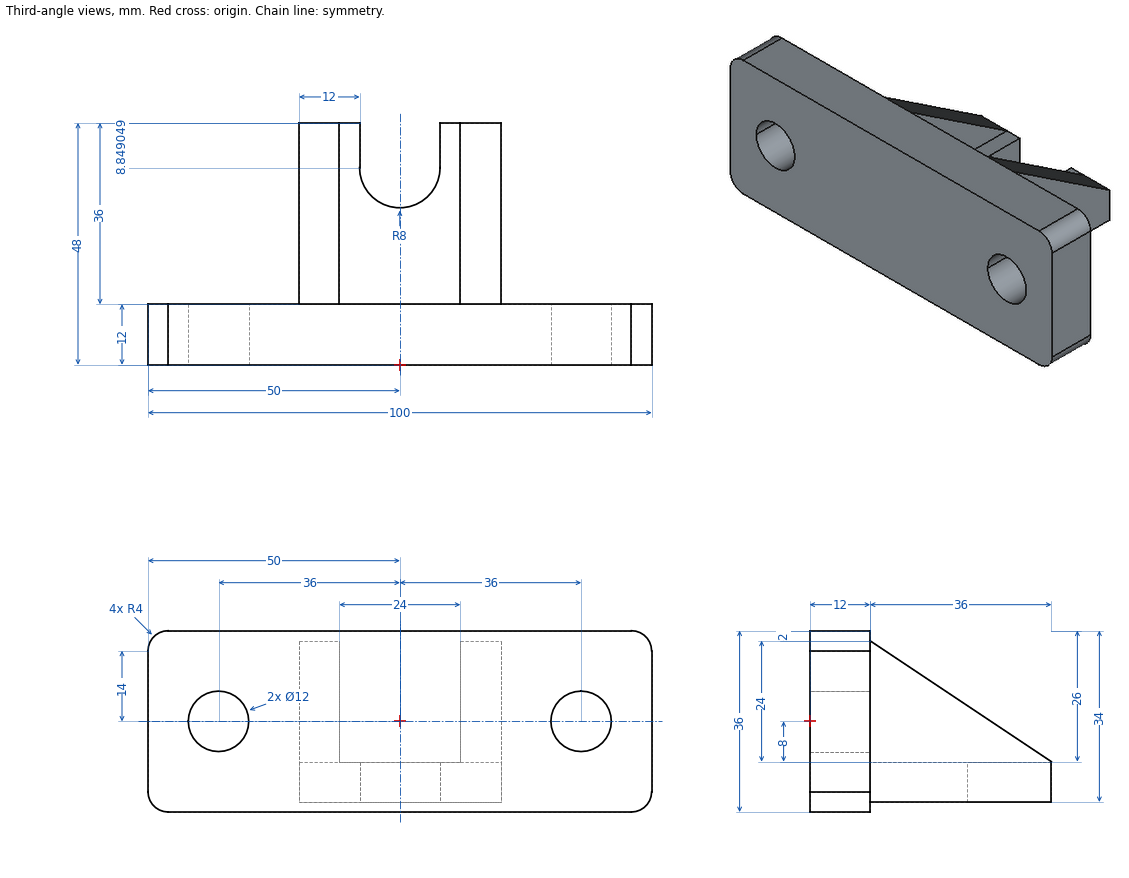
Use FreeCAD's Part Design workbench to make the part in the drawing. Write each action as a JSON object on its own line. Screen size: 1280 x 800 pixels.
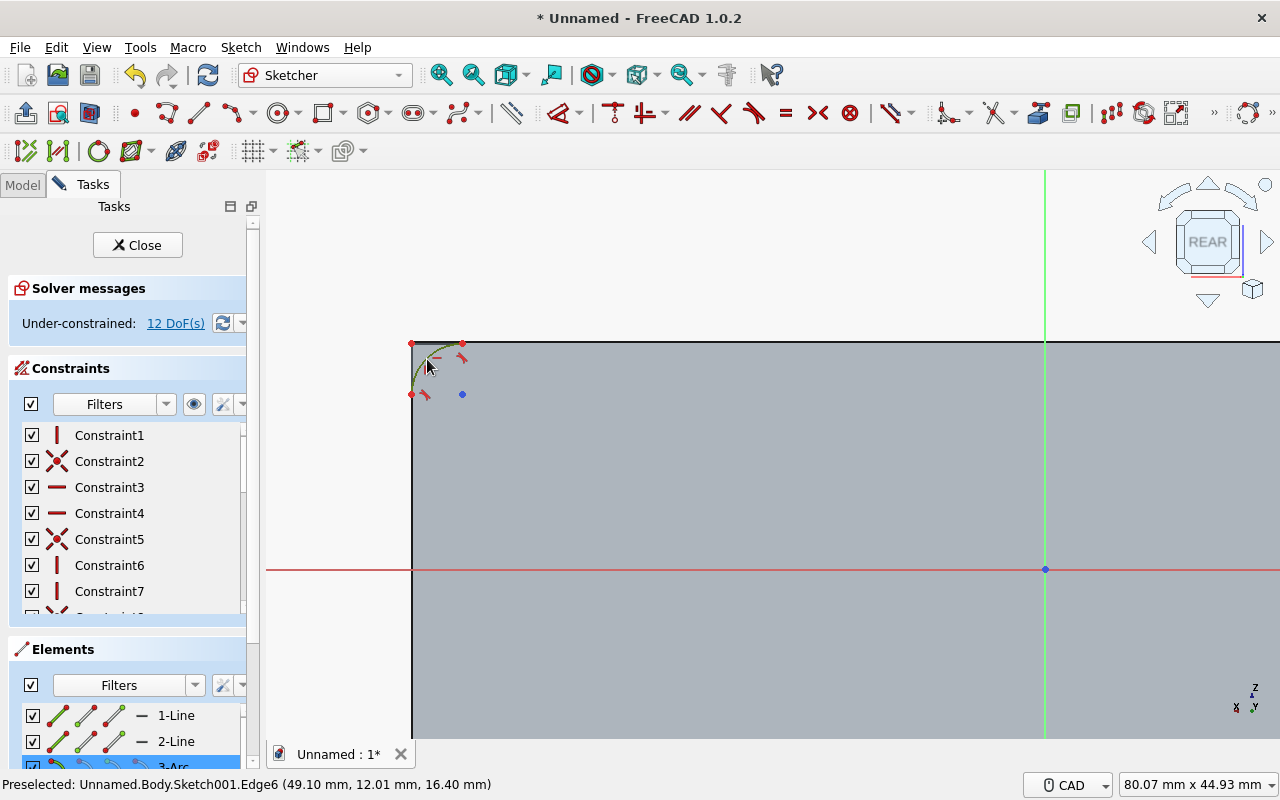
{"action": "scroll", "coordinate": [426, 360], "scroll_direction": "down", "scroll_amount": 4}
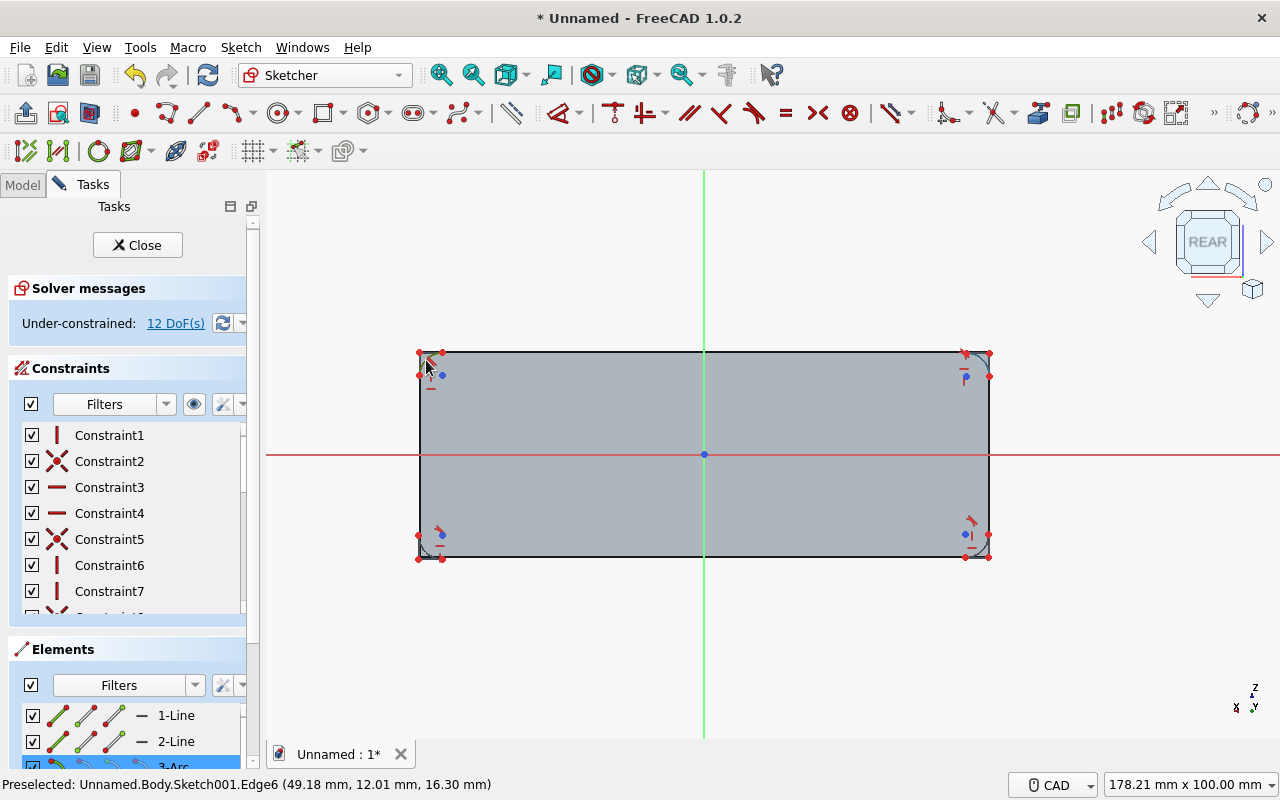
{"action": "scroll", "coordinate": [426, 552], "scroll_direction": "up", "scroll_amount": 4}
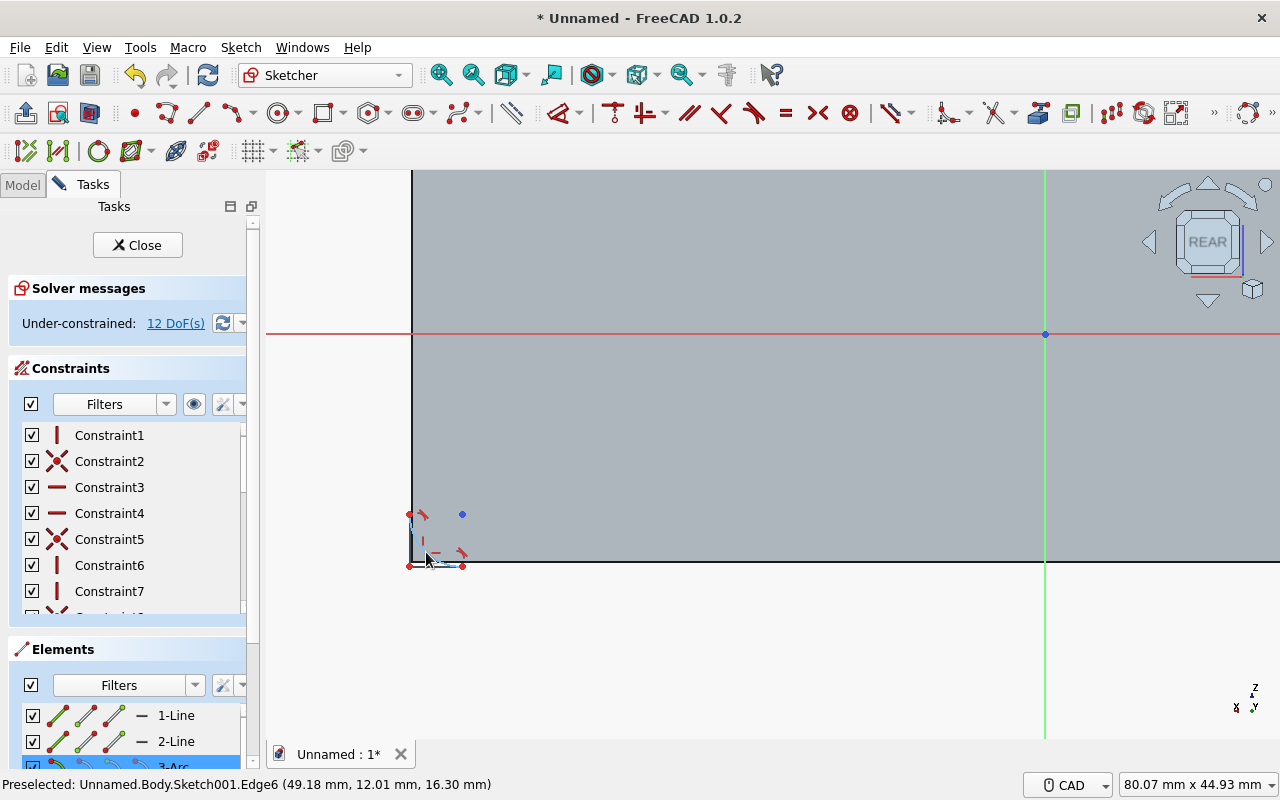
{"action": "left_click", "coordinate": [425, 551]}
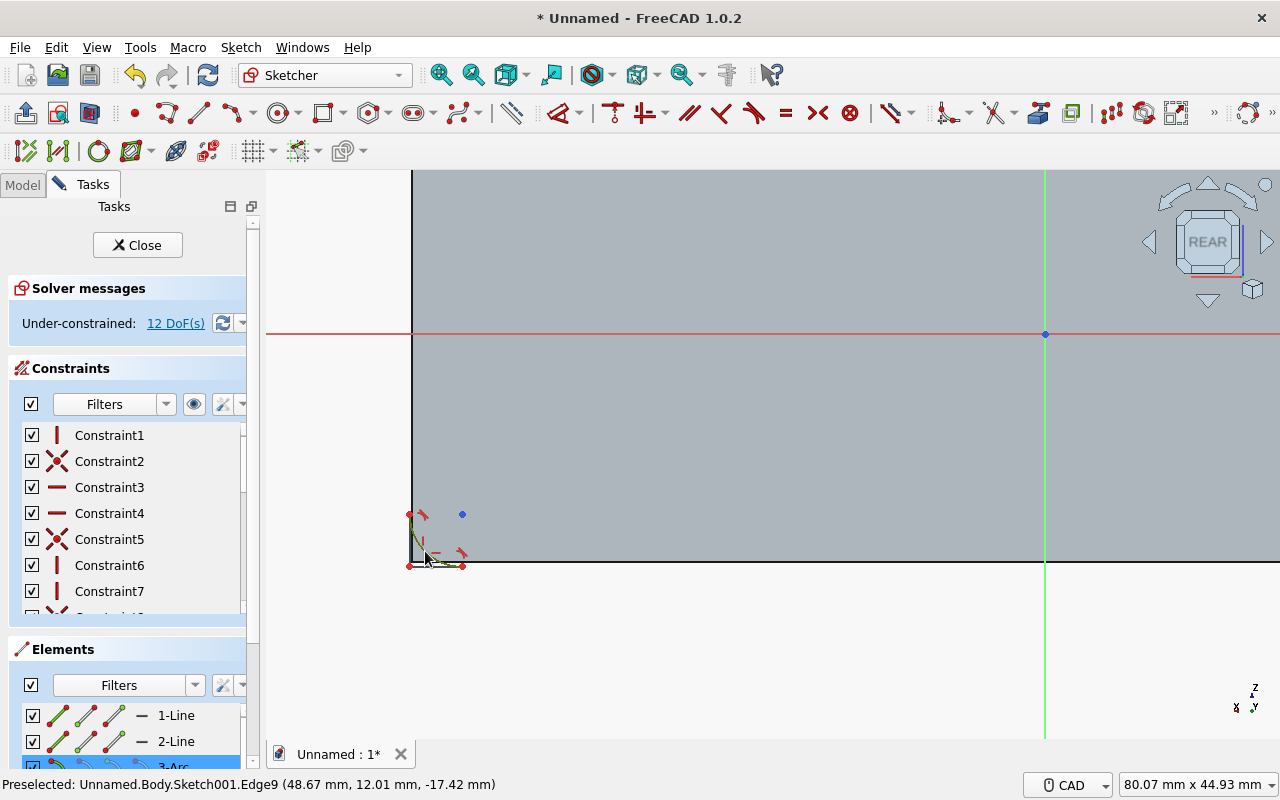
{"action": "scroll", "coordinate": [426, 553], "scroll_direction": "down", "scroll_amount": 4}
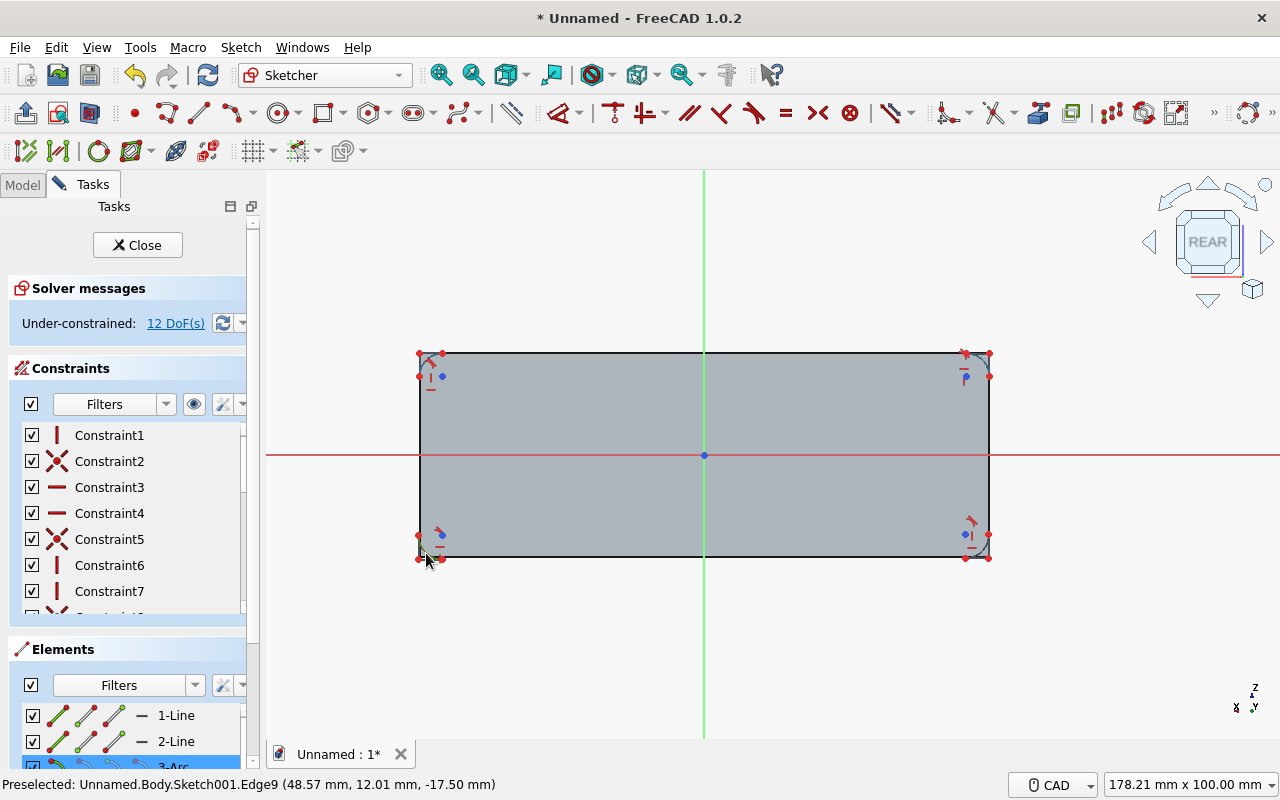
{"action": "scroll", "coordinate": [982, 551], "scroll_direction": "up", "scroll_amount": 4}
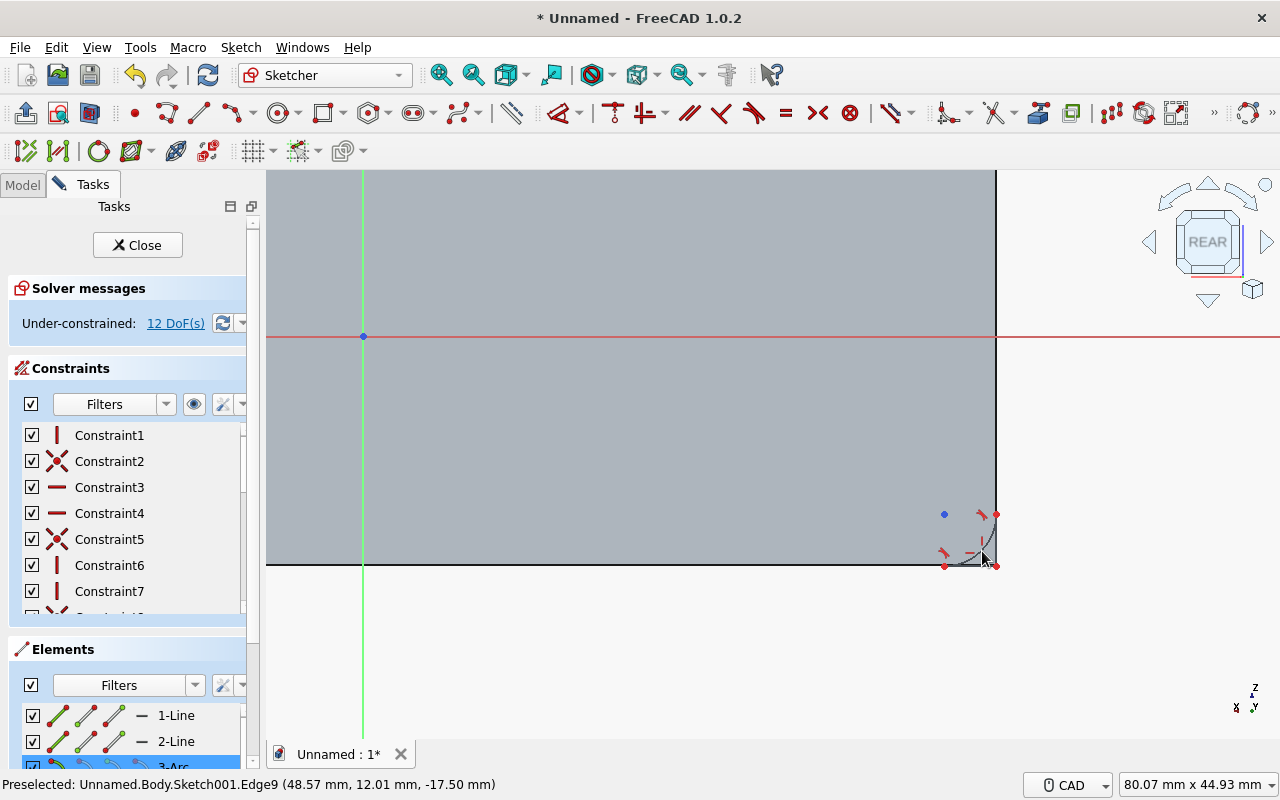
{"action": "left_click", "coordinate": [981, 551]}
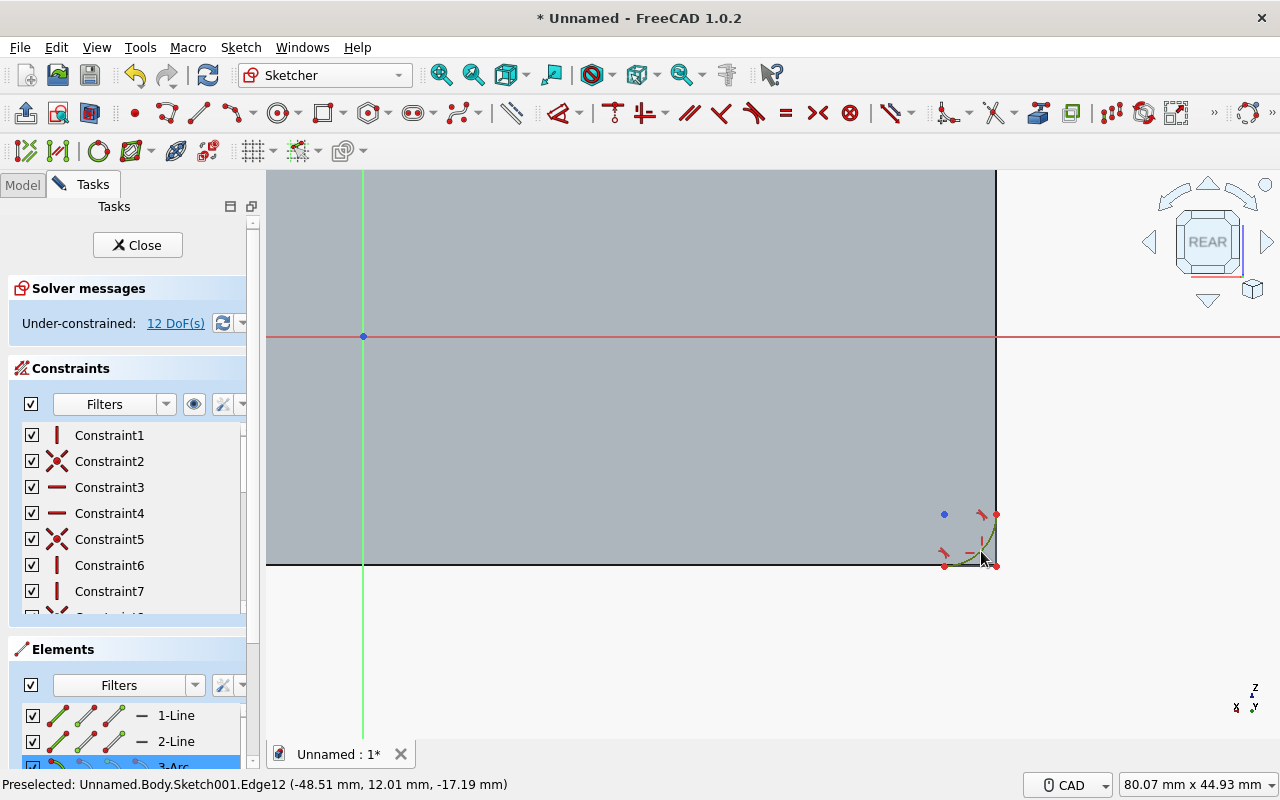
{"action": "left_click", "coordinate": [786, 114]}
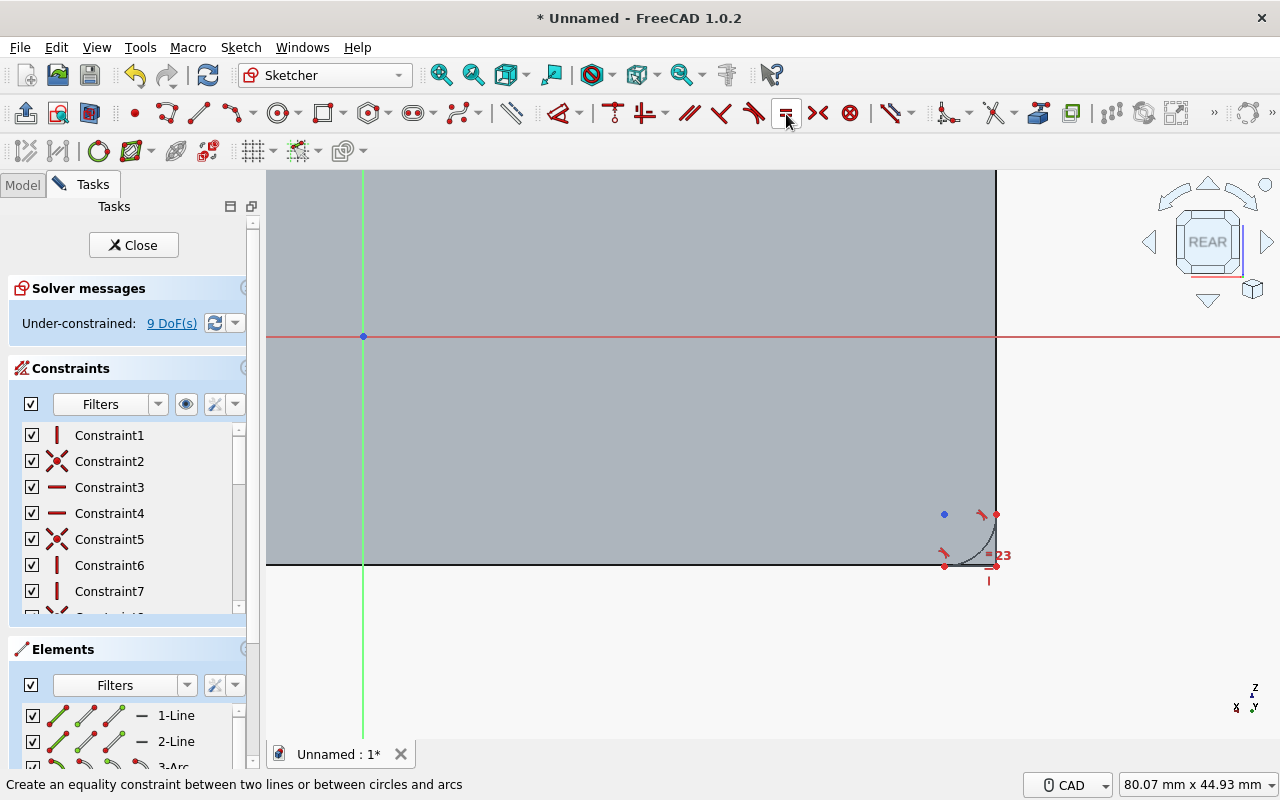
{"action": "scroll", "coordinate": [983, 551], "scroll_direction": "down", "scroll_amount": 4}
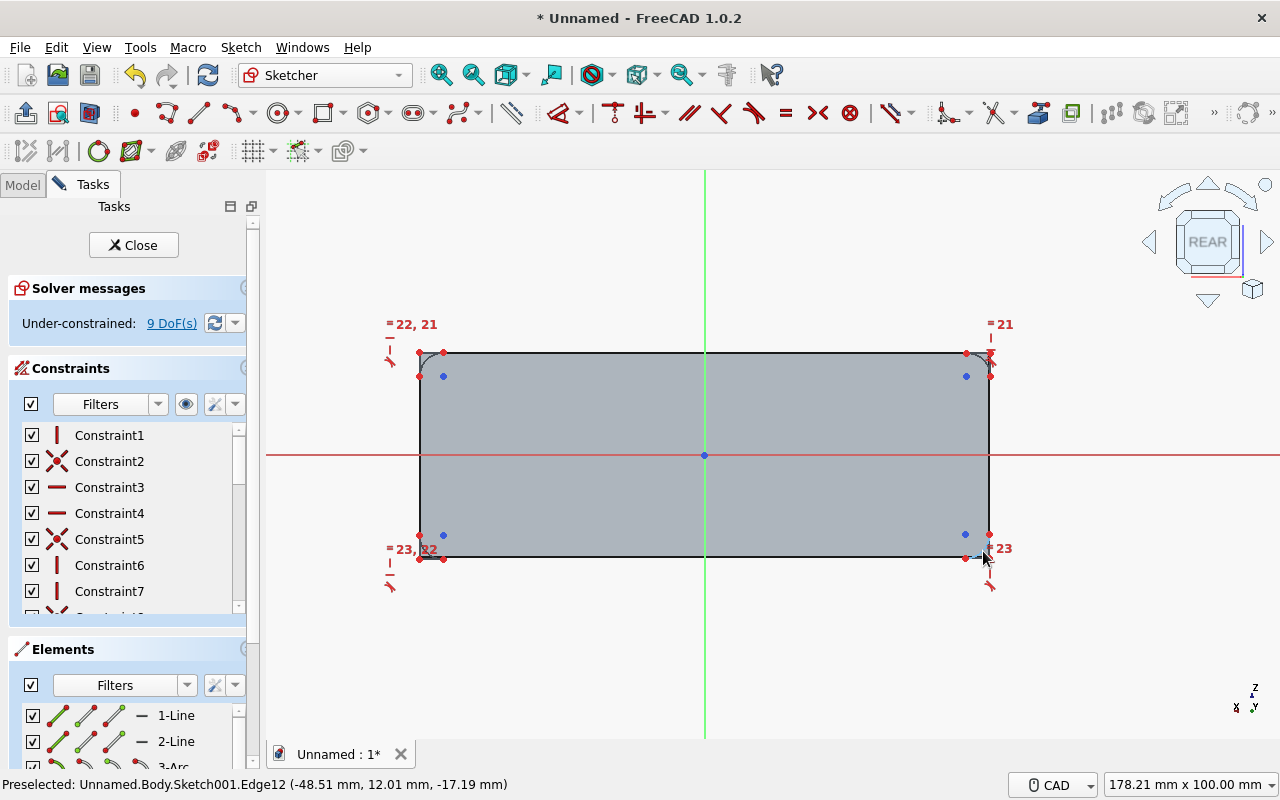
{"action": "left_click", "coordinate": [967, 377]}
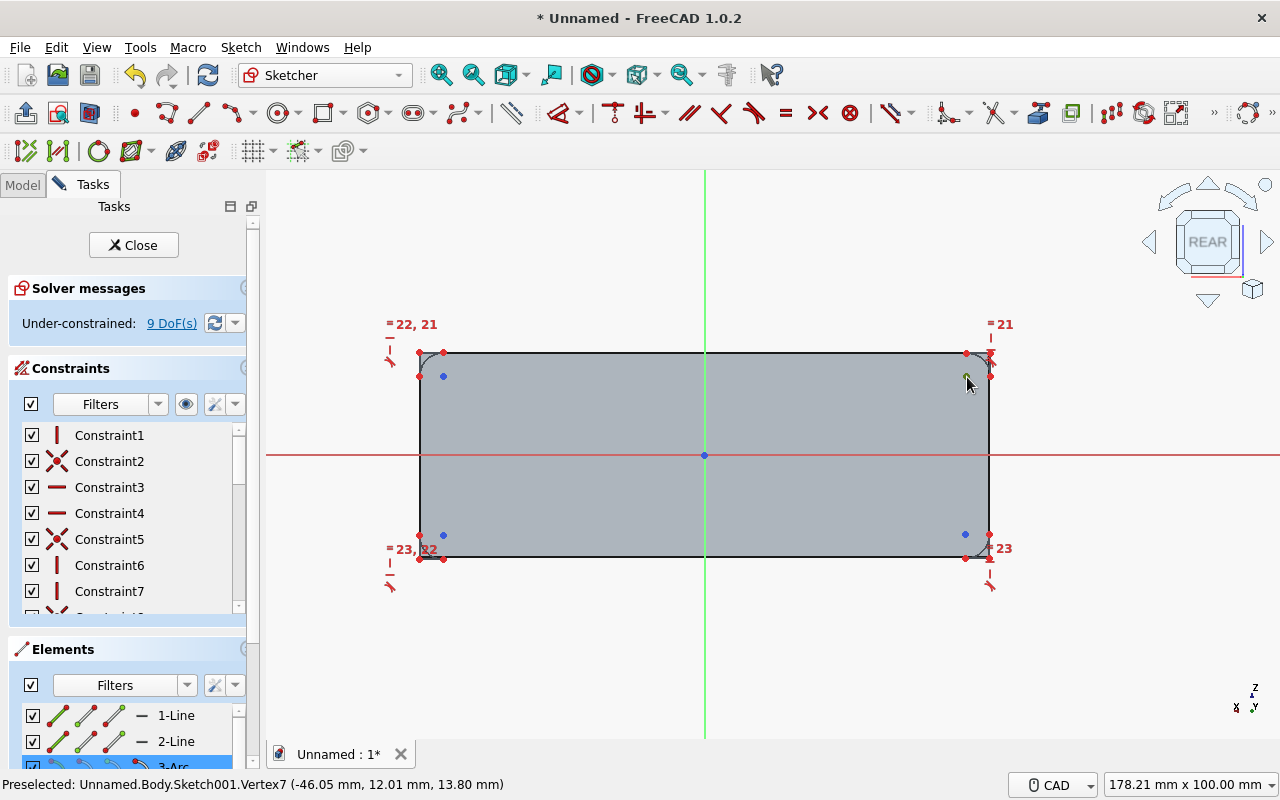
{"action": "left_click", "coordinate": [443, 376]}